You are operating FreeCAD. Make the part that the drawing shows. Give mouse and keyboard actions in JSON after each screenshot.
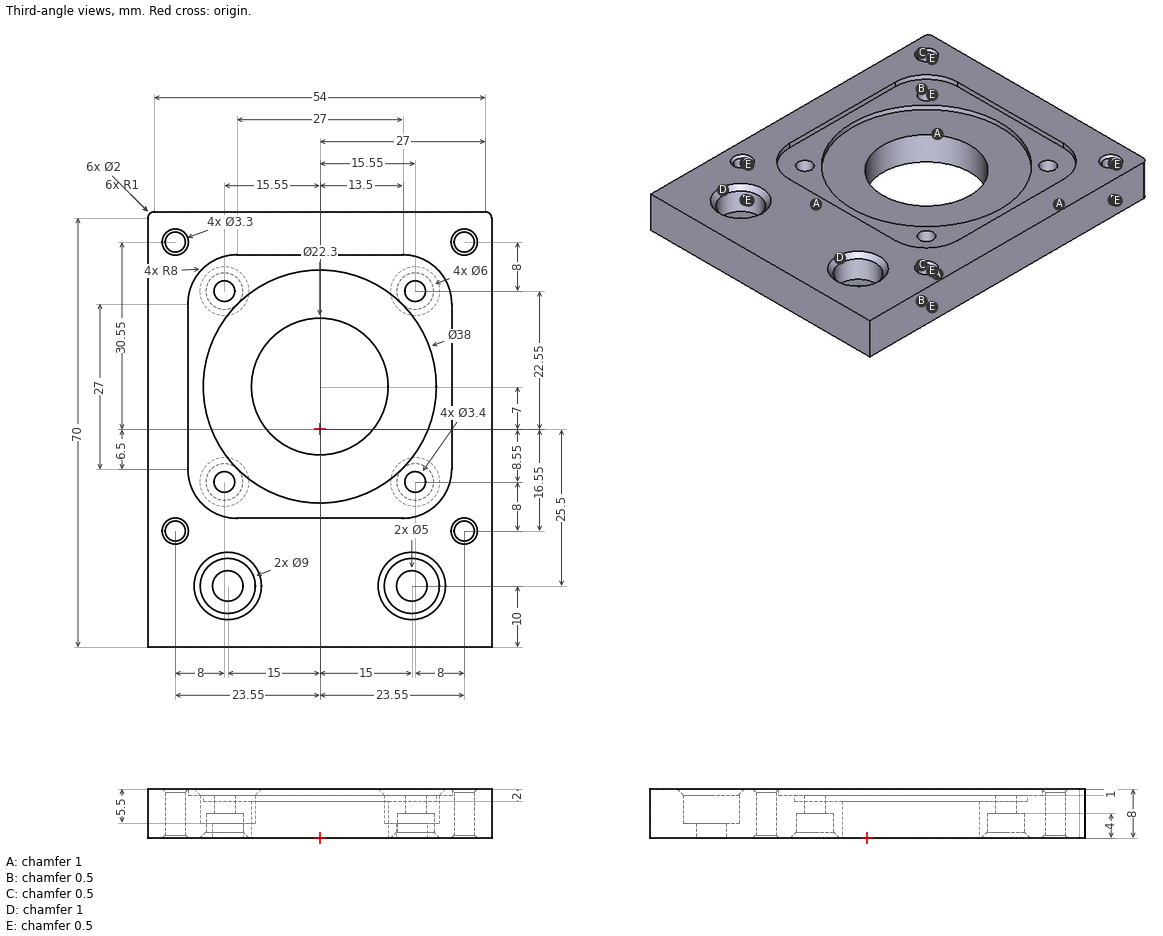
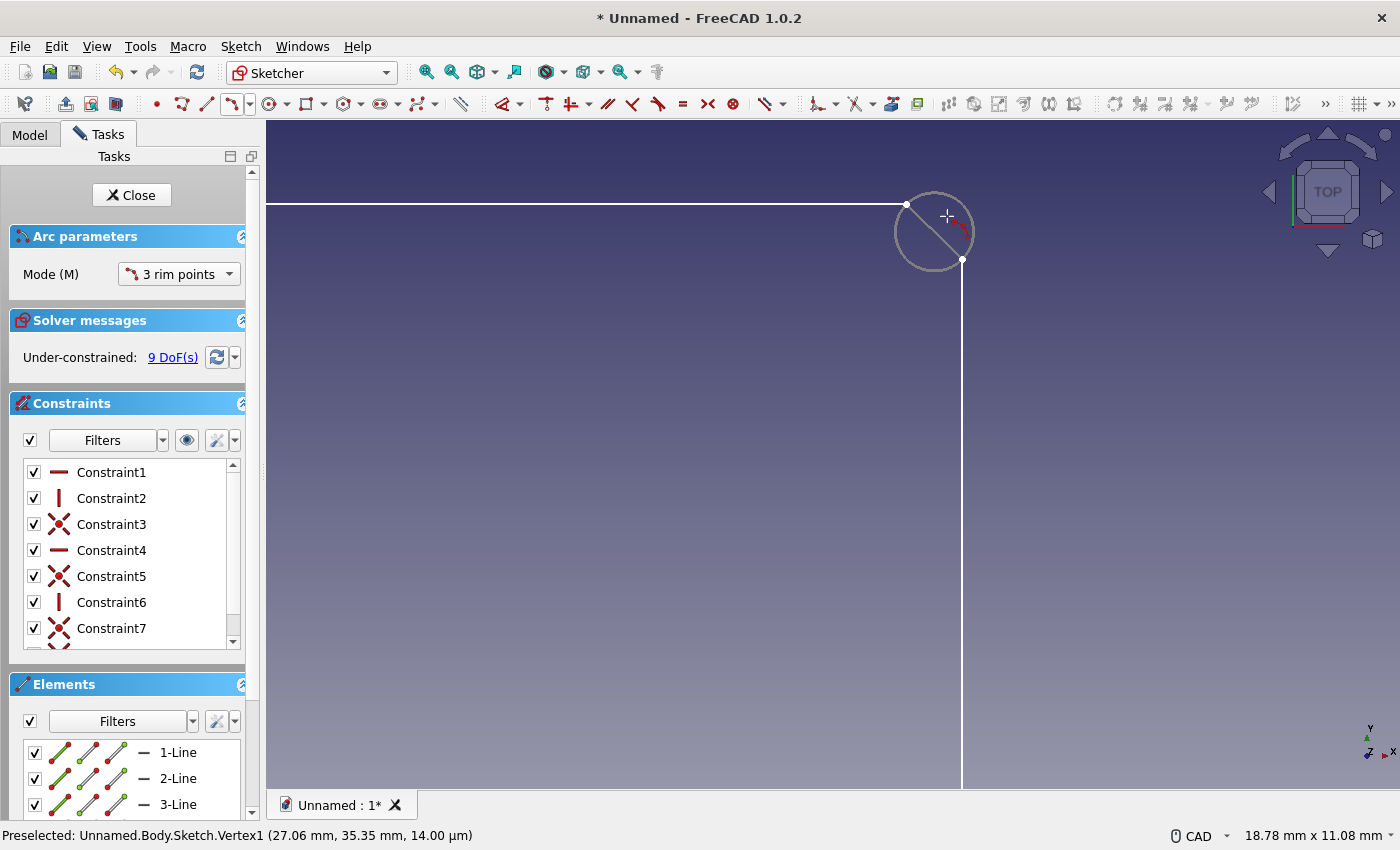
{"action": "left_click", "coordinate": [946, 213]}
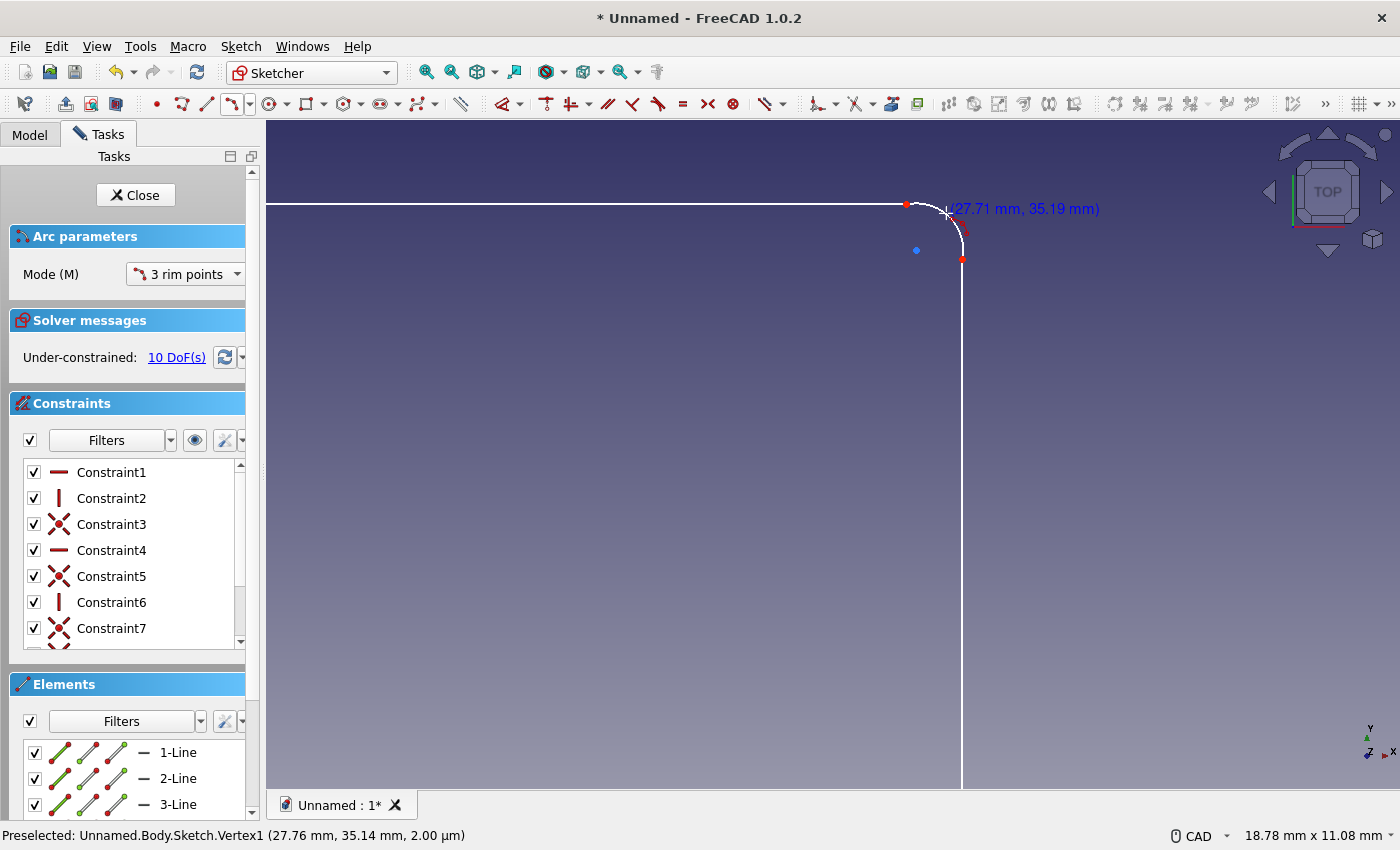
{"action": "left_click", "coordinate": [268, 104]}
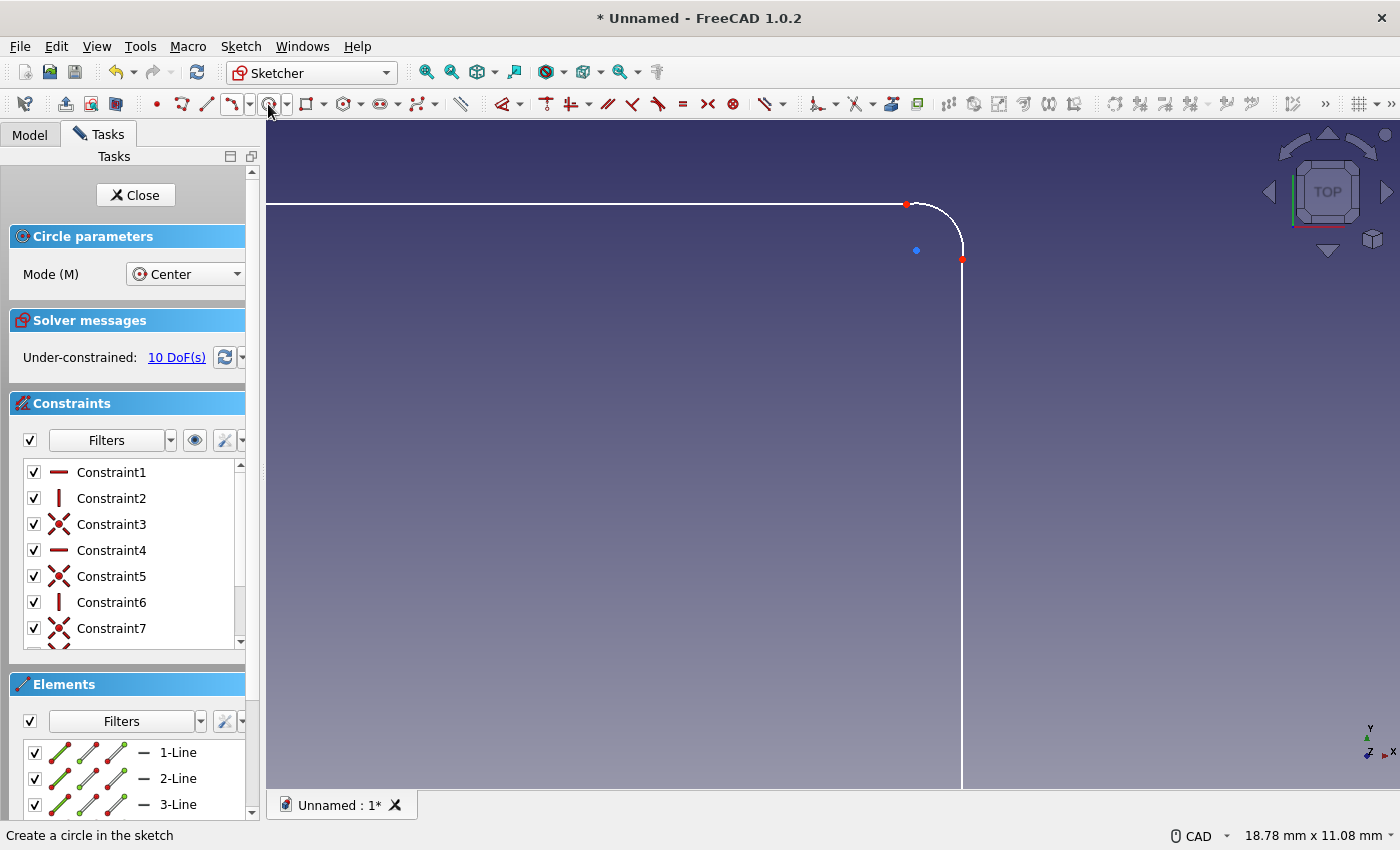
{"action": "scroll", "coordinate": [950, 220], "scroll_direction": "down", "scroll_amount": 11}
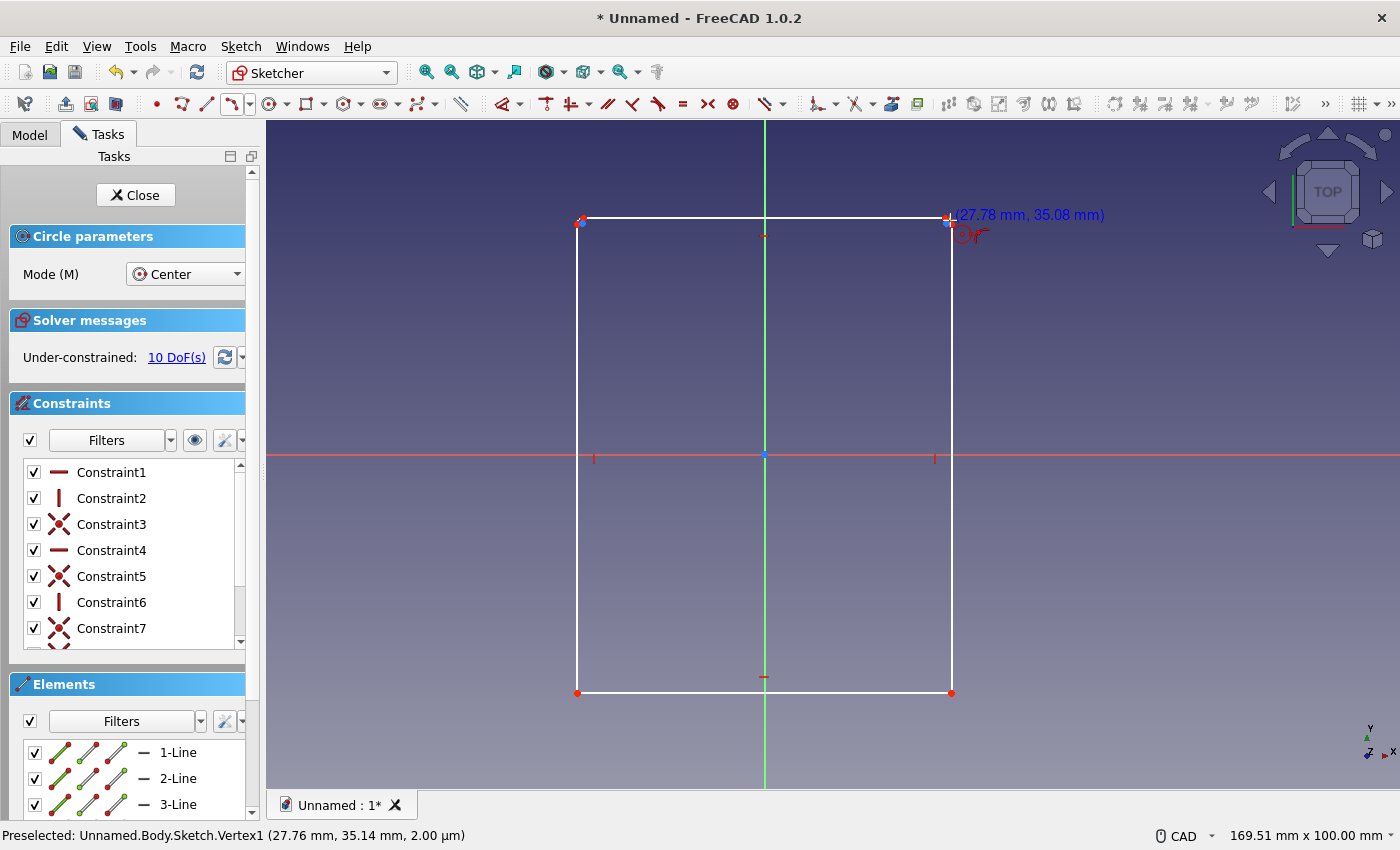
{"action": "scroll", "coordinate": [865, 626], "scroll_direction": "up", "scroll_amount": 2}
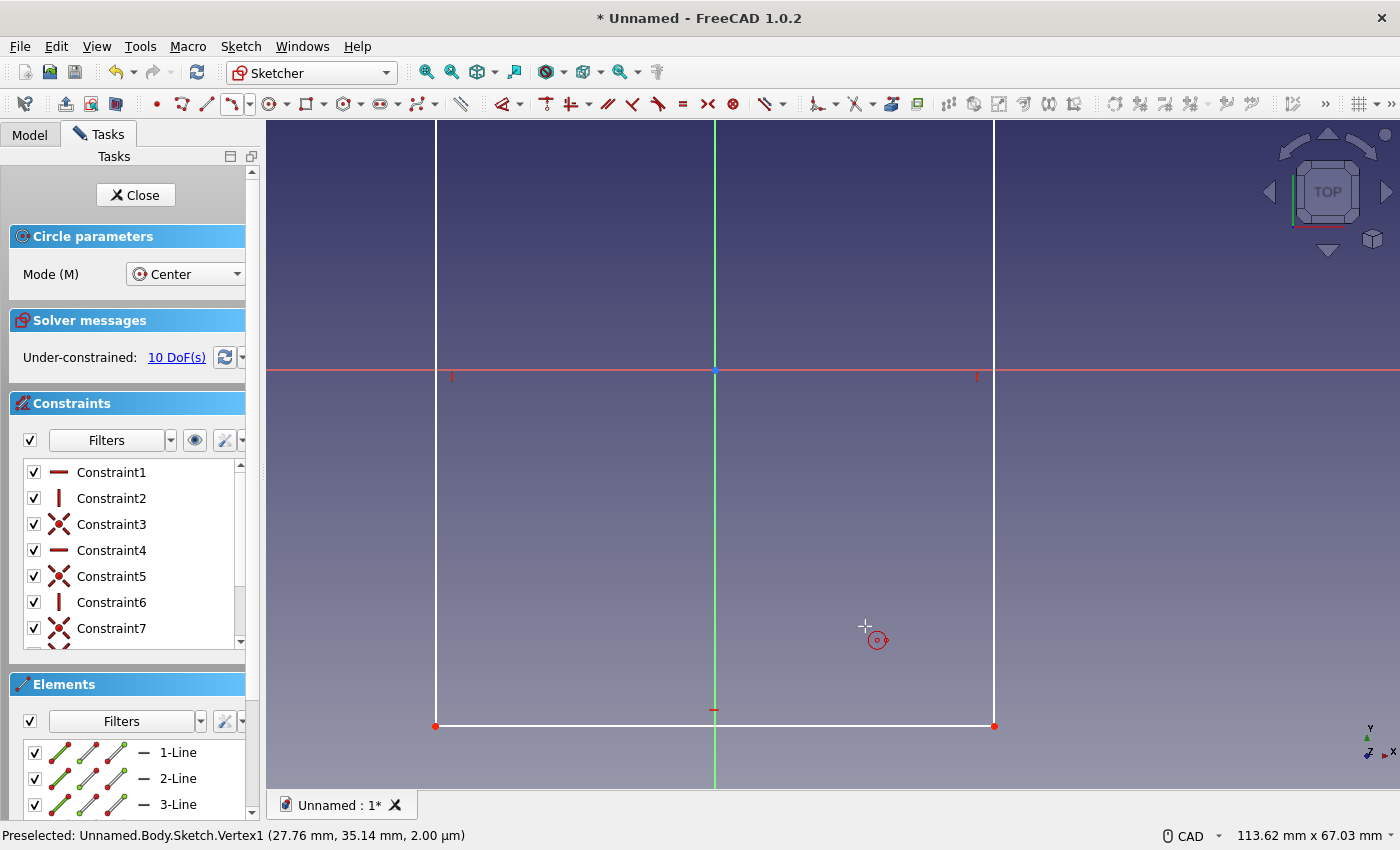
{"action": "left_click", "coordinate": [865, 625]}
{"action": "left_click", "coordinate": [882, 607]}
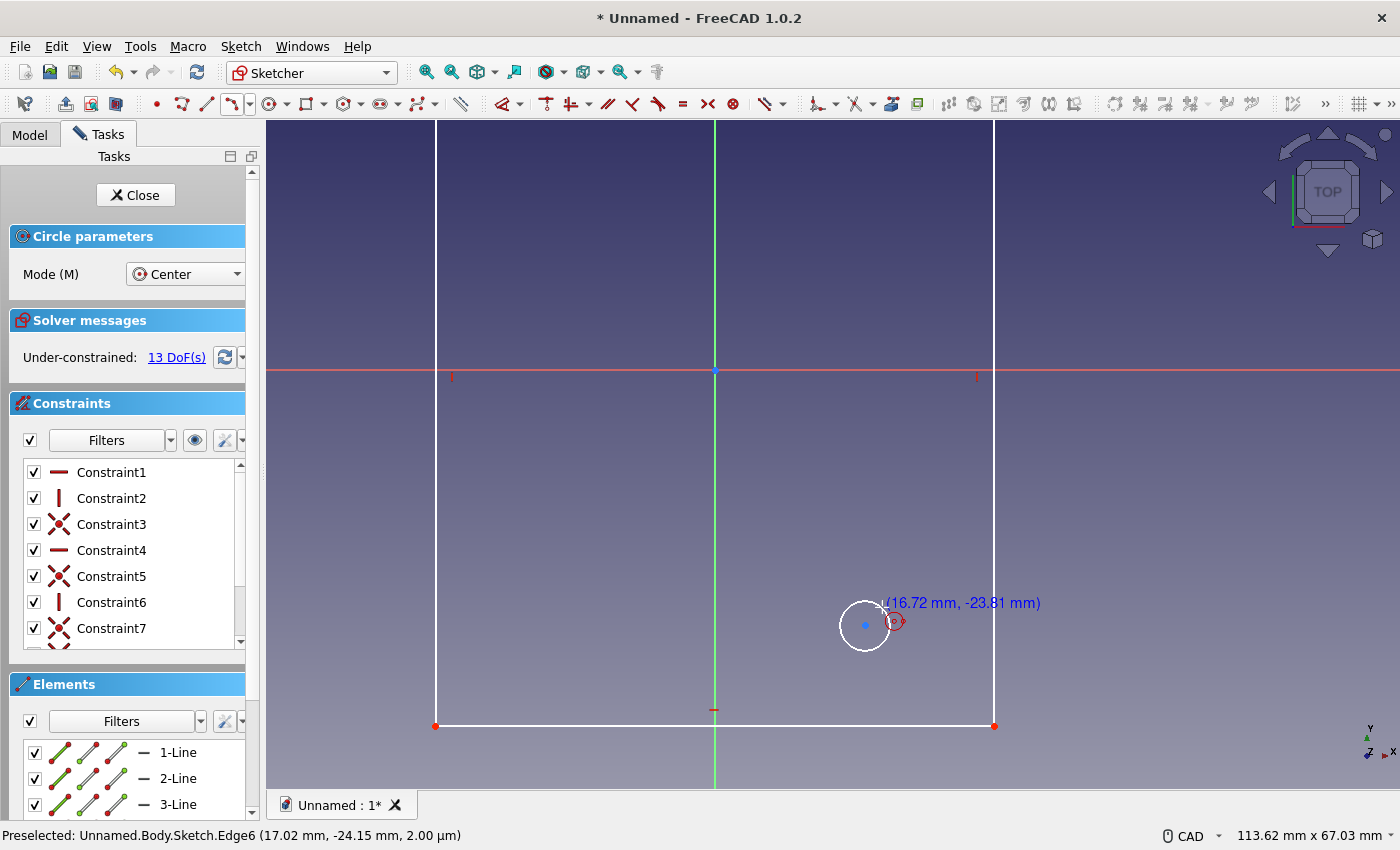
{"action": "scroll", "coordinate": [950, 536], "scroll_direction": "up", "scroll_amount": 5}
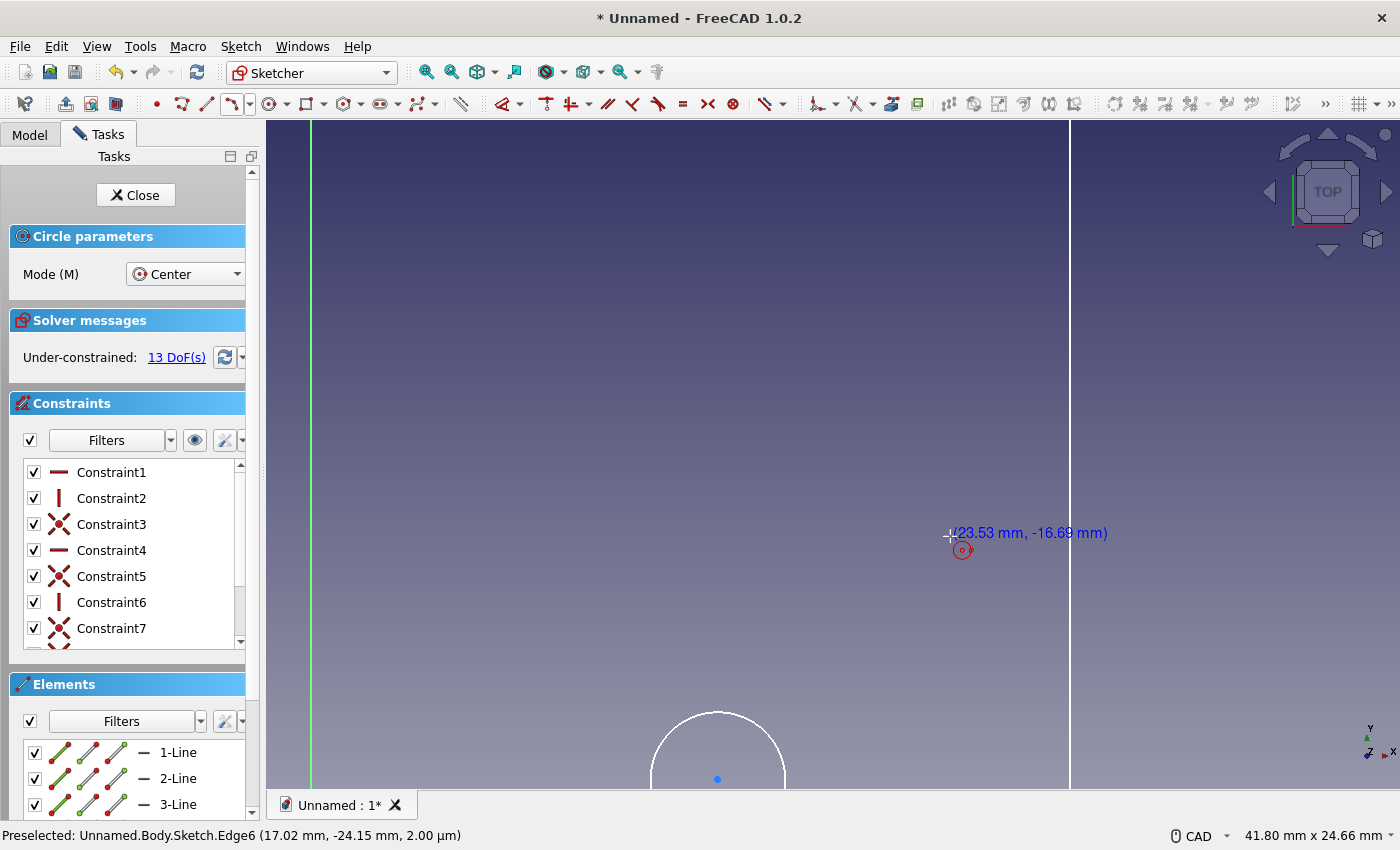
{"action": "scroll", "coordinate": [913, 576], "scroll_direction": "down", "scroll_amount": 7}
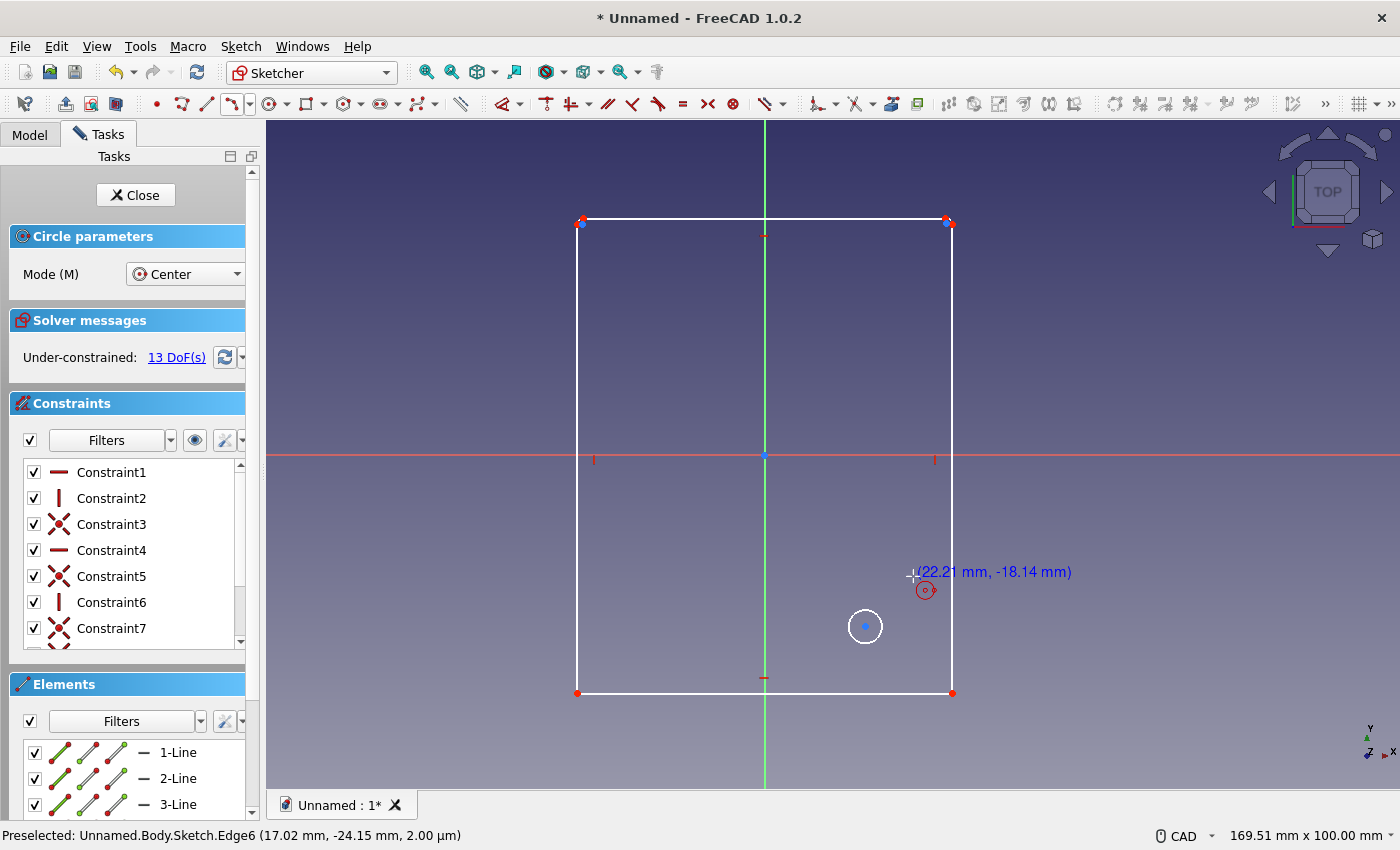
{"action": "left_click", "coordinate": [922, 566]}